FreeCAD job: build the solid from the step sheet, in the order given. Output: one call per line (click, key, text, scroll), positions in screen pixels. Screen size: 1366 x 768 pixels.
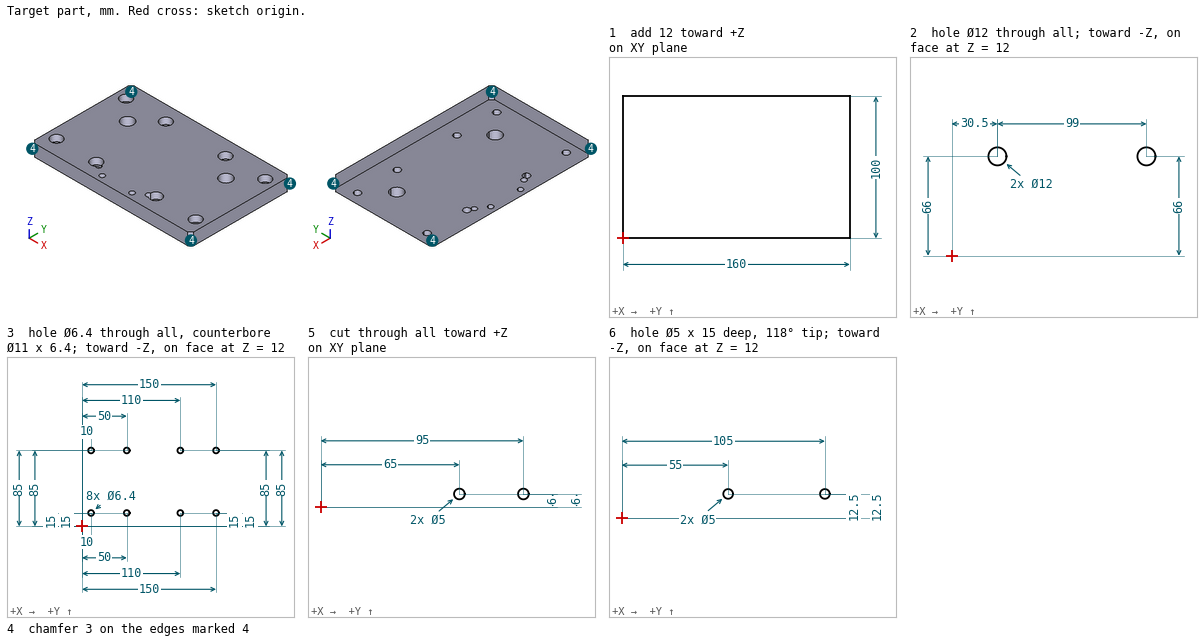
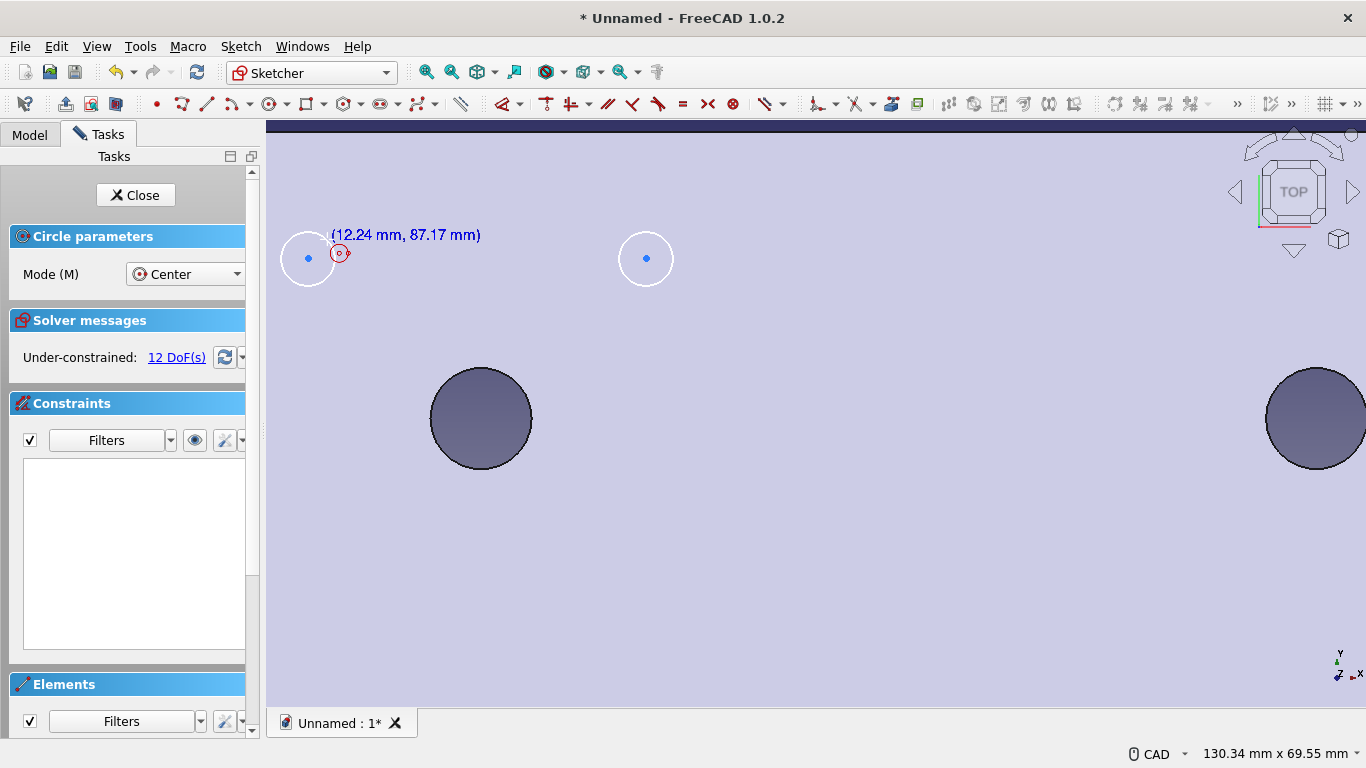
scroll(647, 258, down, 4)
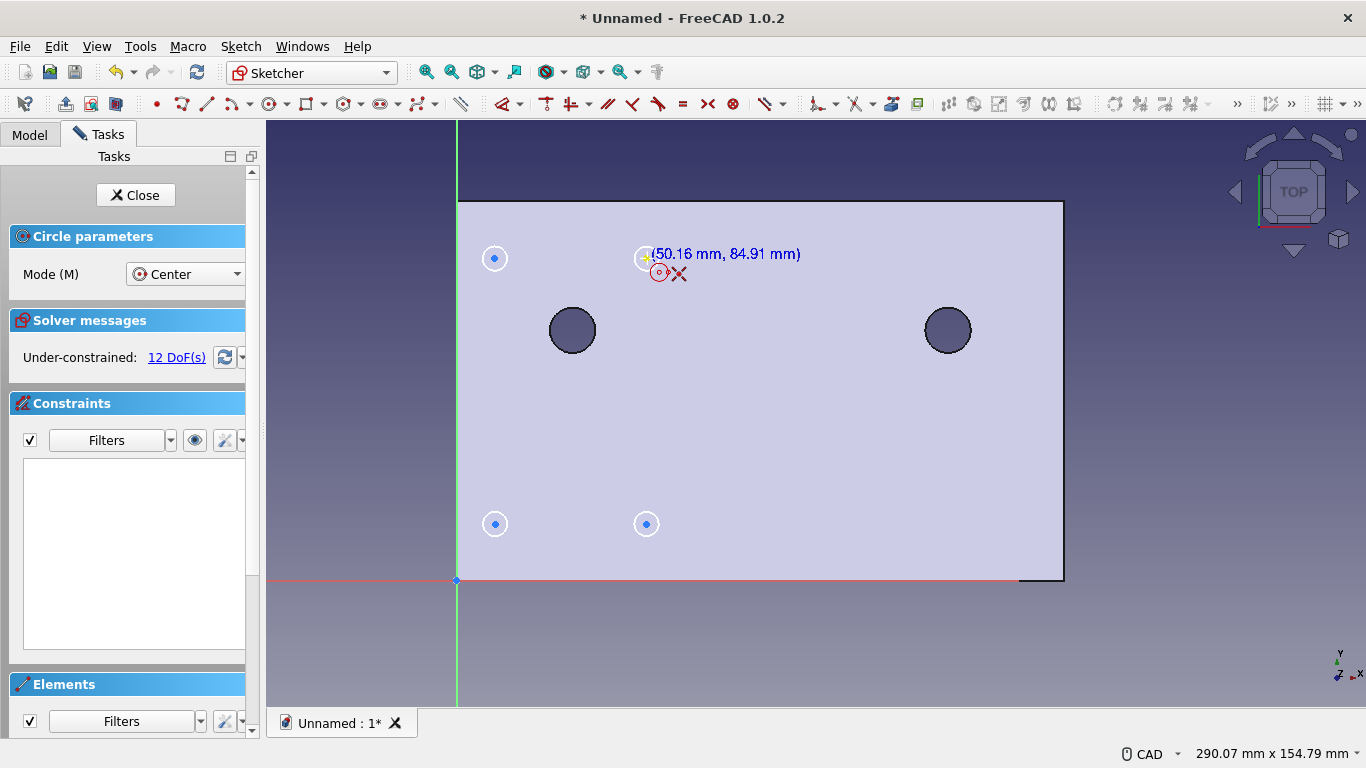
scroll(874, 524, up, 4)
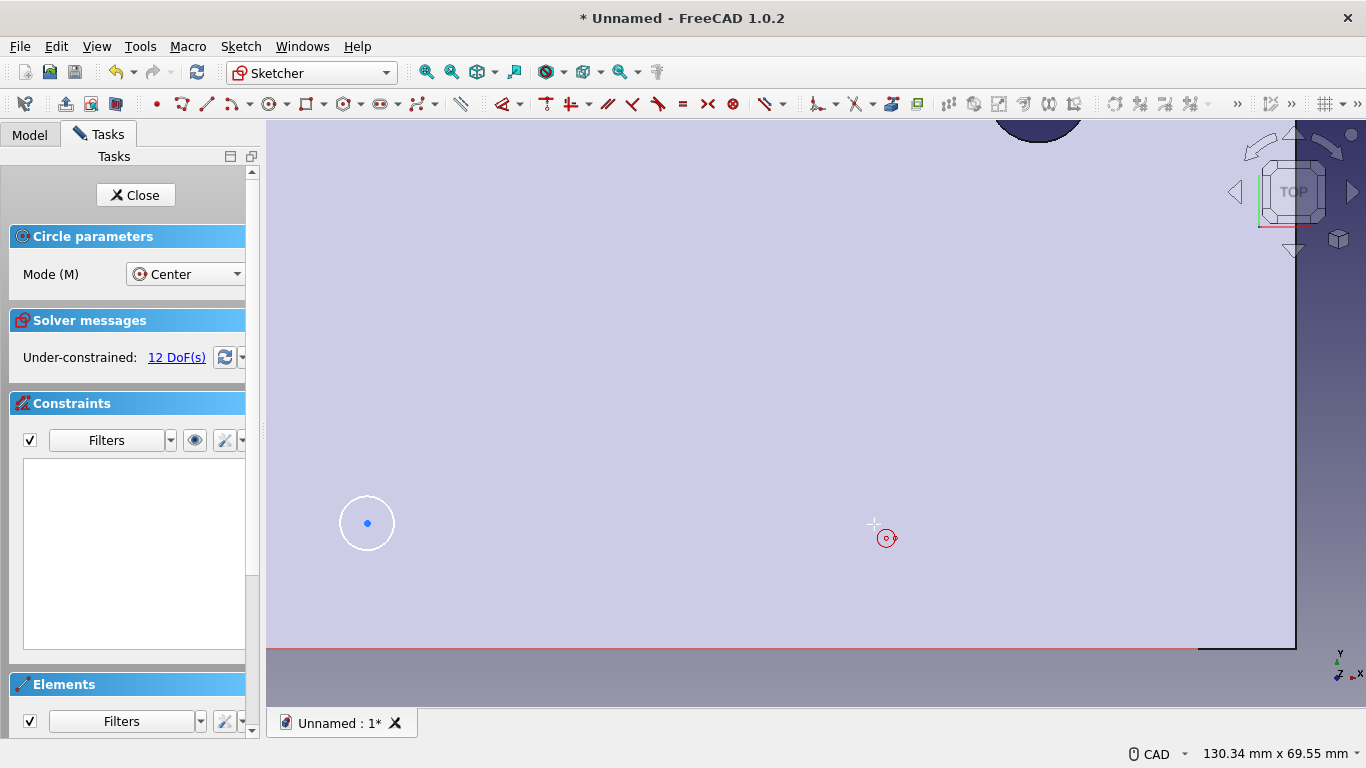
click(874, 523)
click(893, 503)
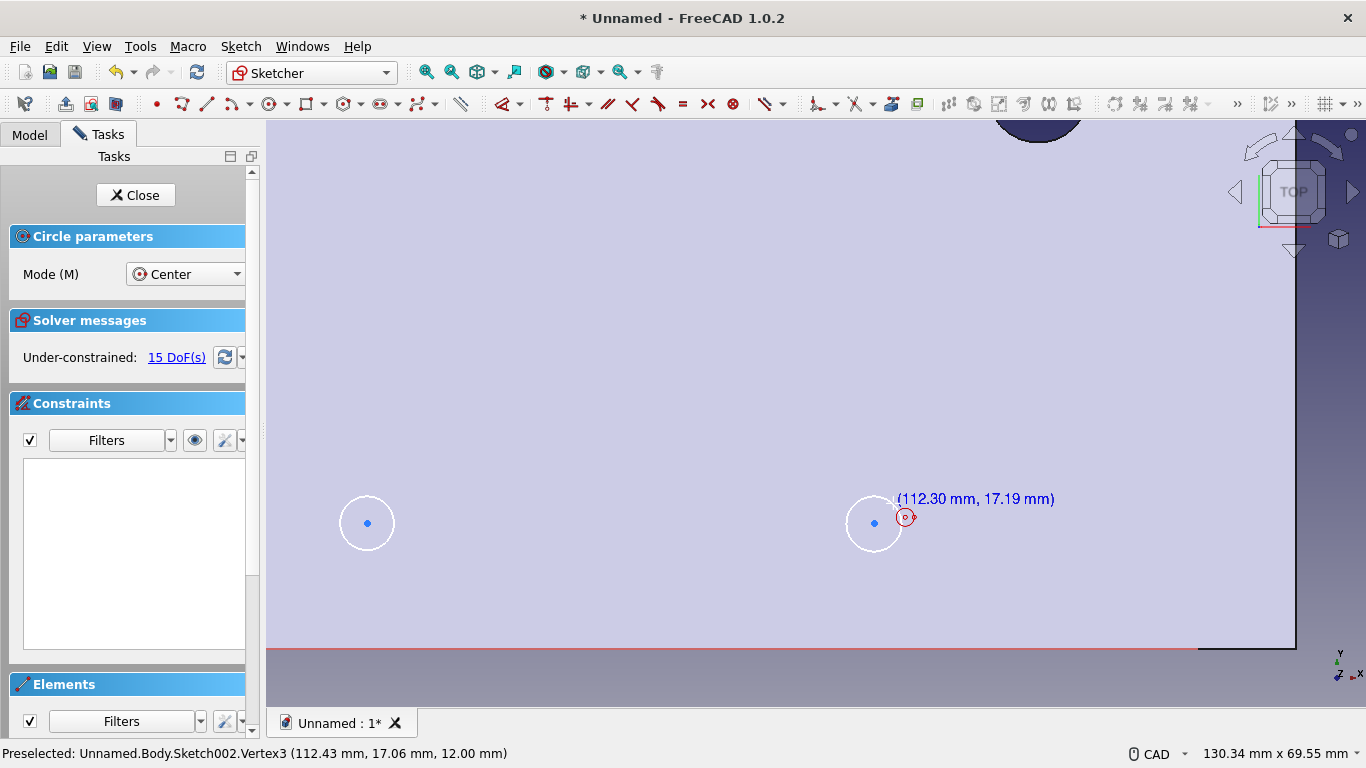
scroll(875, 525, down, 4)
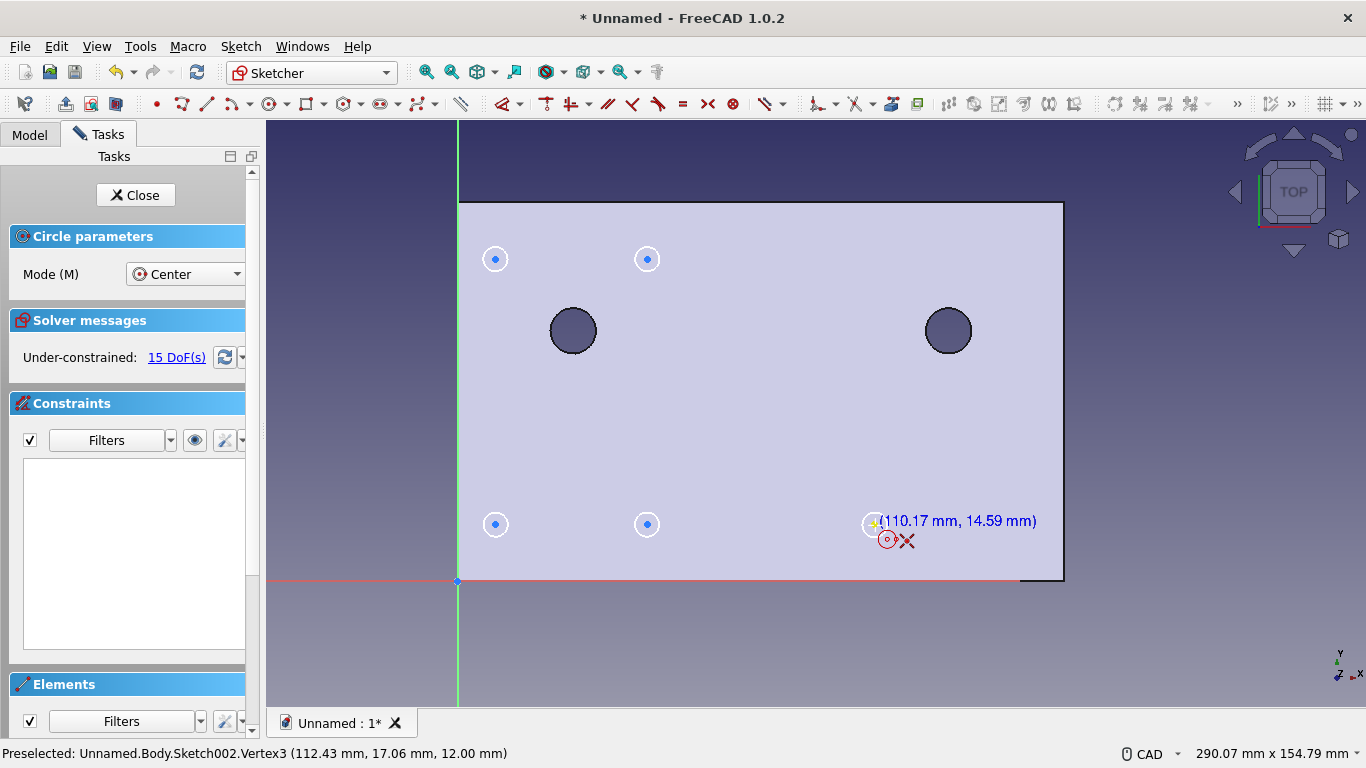
scroll(1026, 524, up, 4)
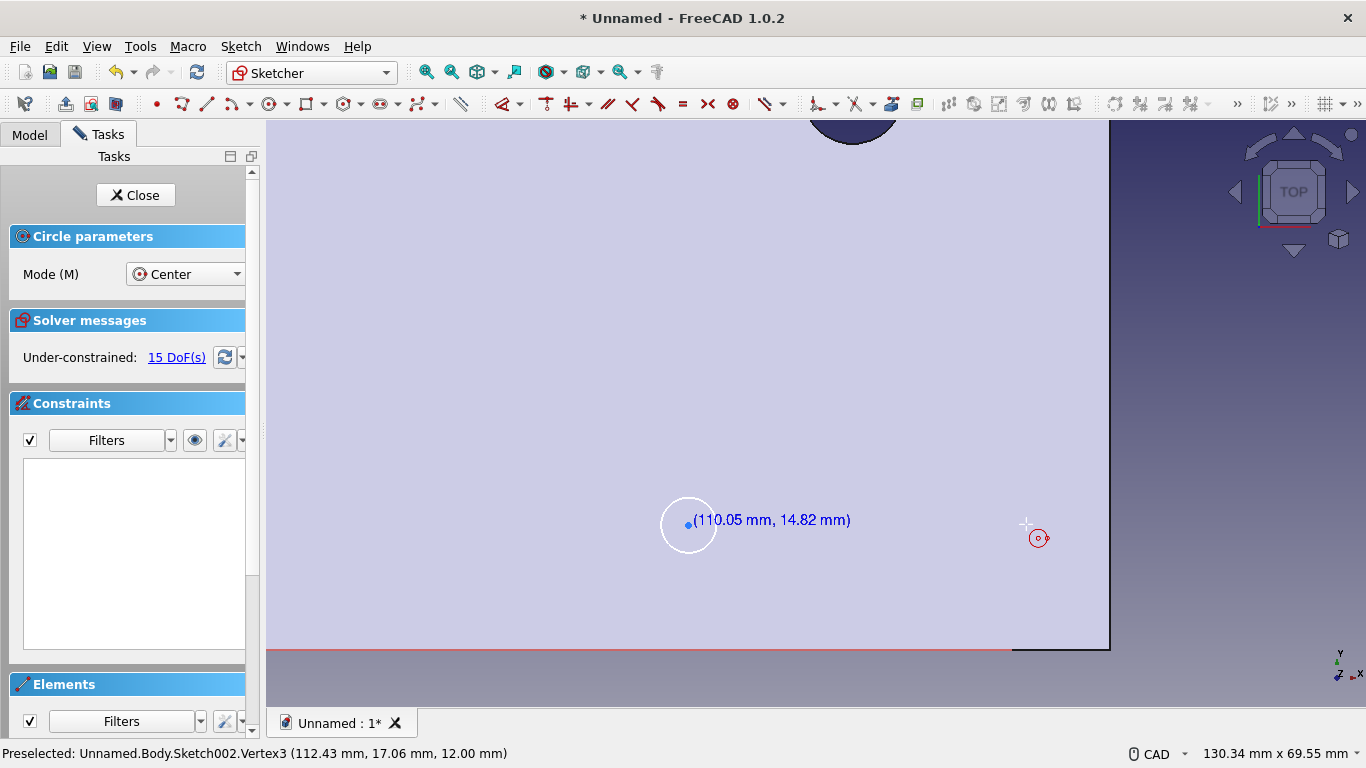
click(1026, 524)
click(1045, 505)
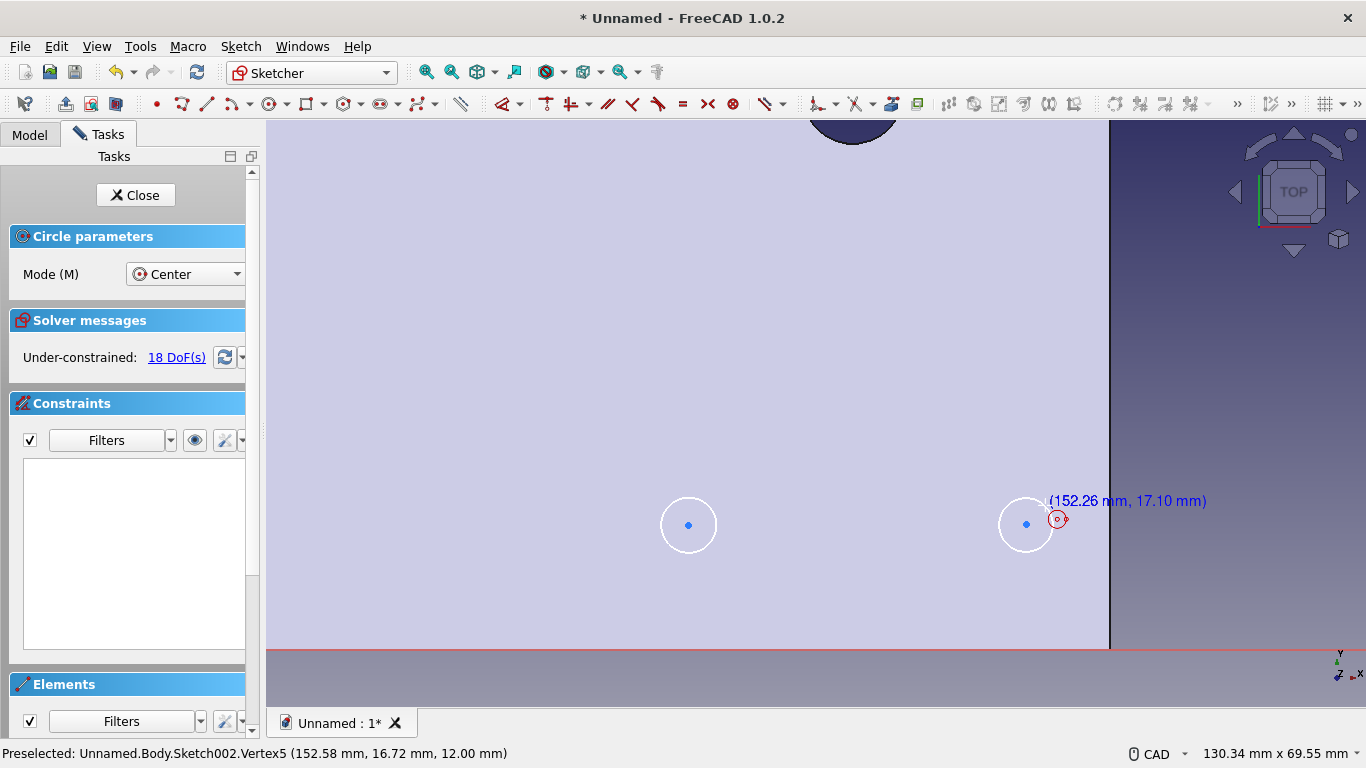
scroll(1026, 524, down, 4)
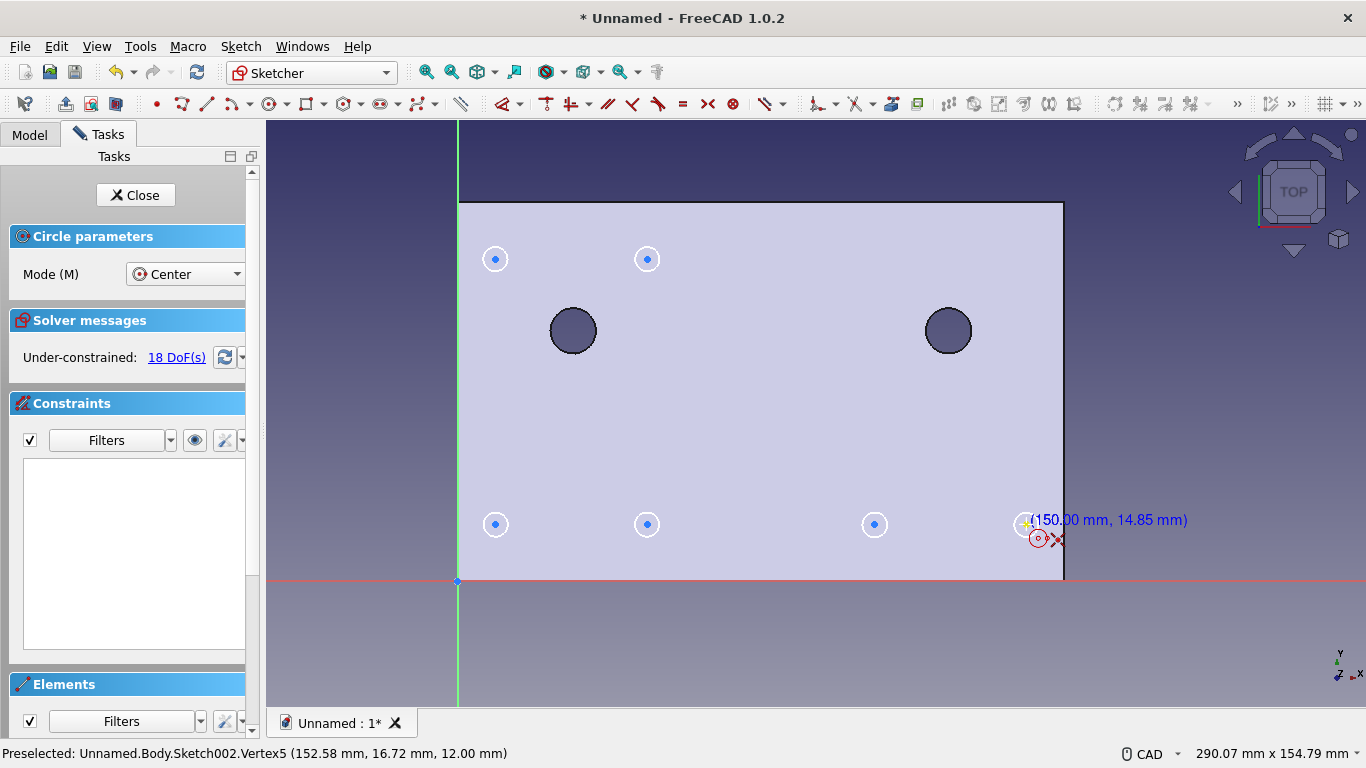
scroll(1026, 259, up, 4)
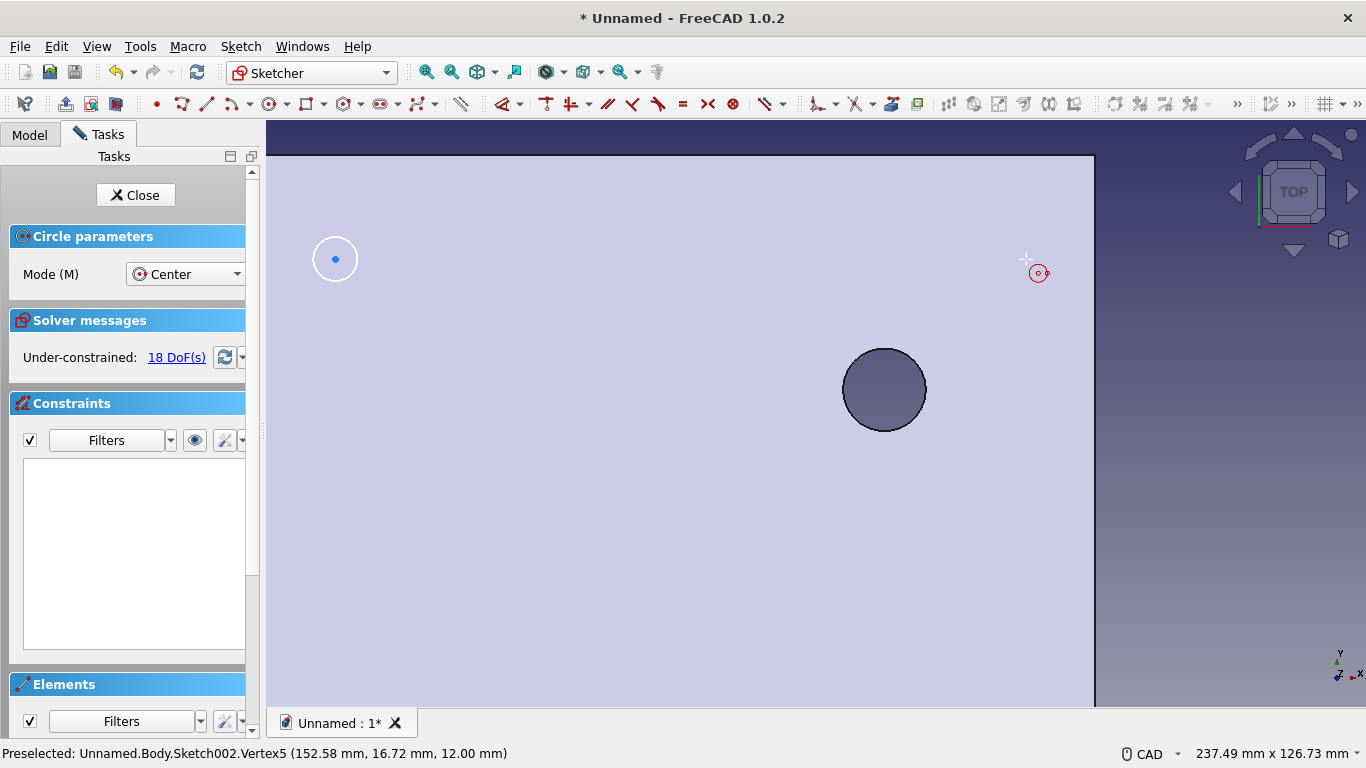
click(1026, 258)
click(1045, 239)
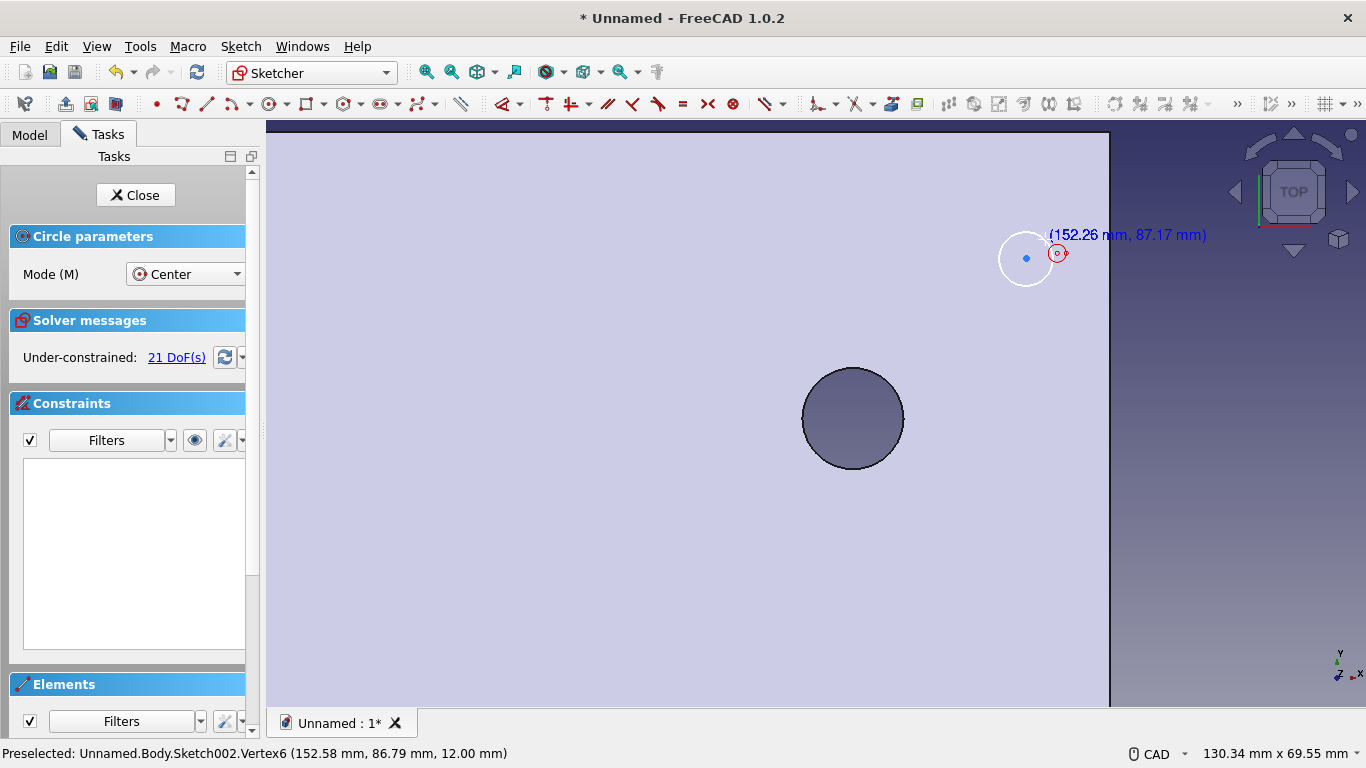
click(688, 258)
click(707, 239)
key(Escape)